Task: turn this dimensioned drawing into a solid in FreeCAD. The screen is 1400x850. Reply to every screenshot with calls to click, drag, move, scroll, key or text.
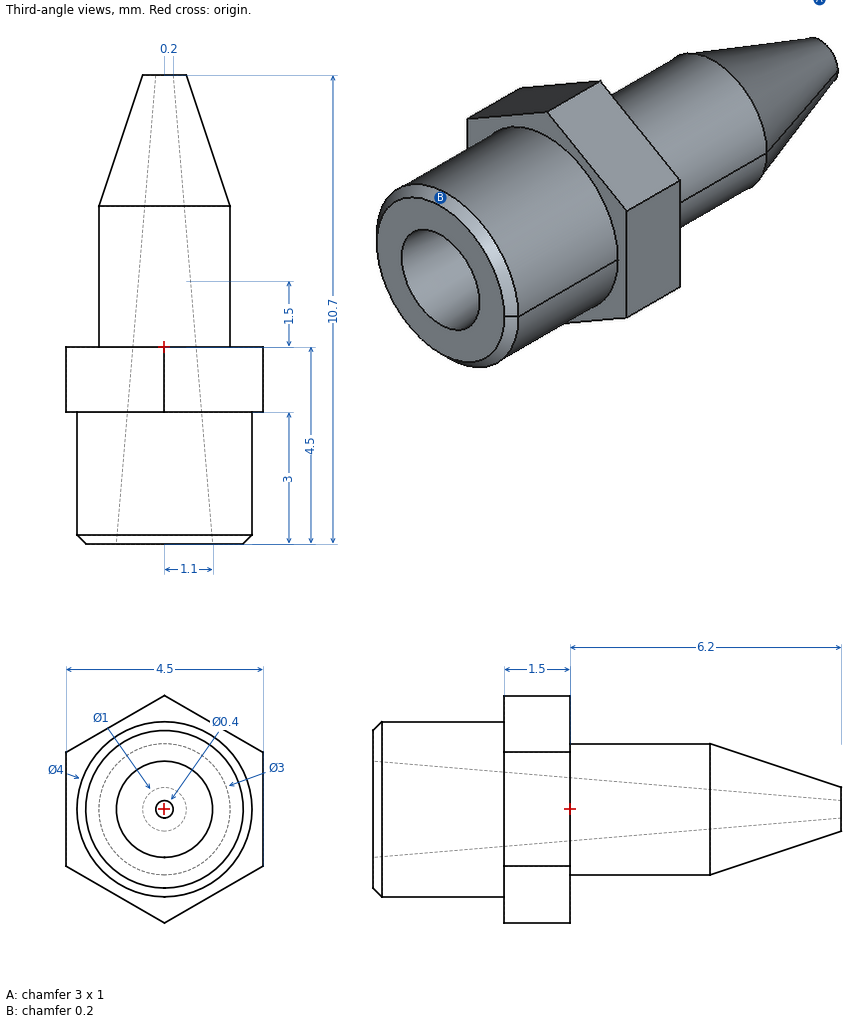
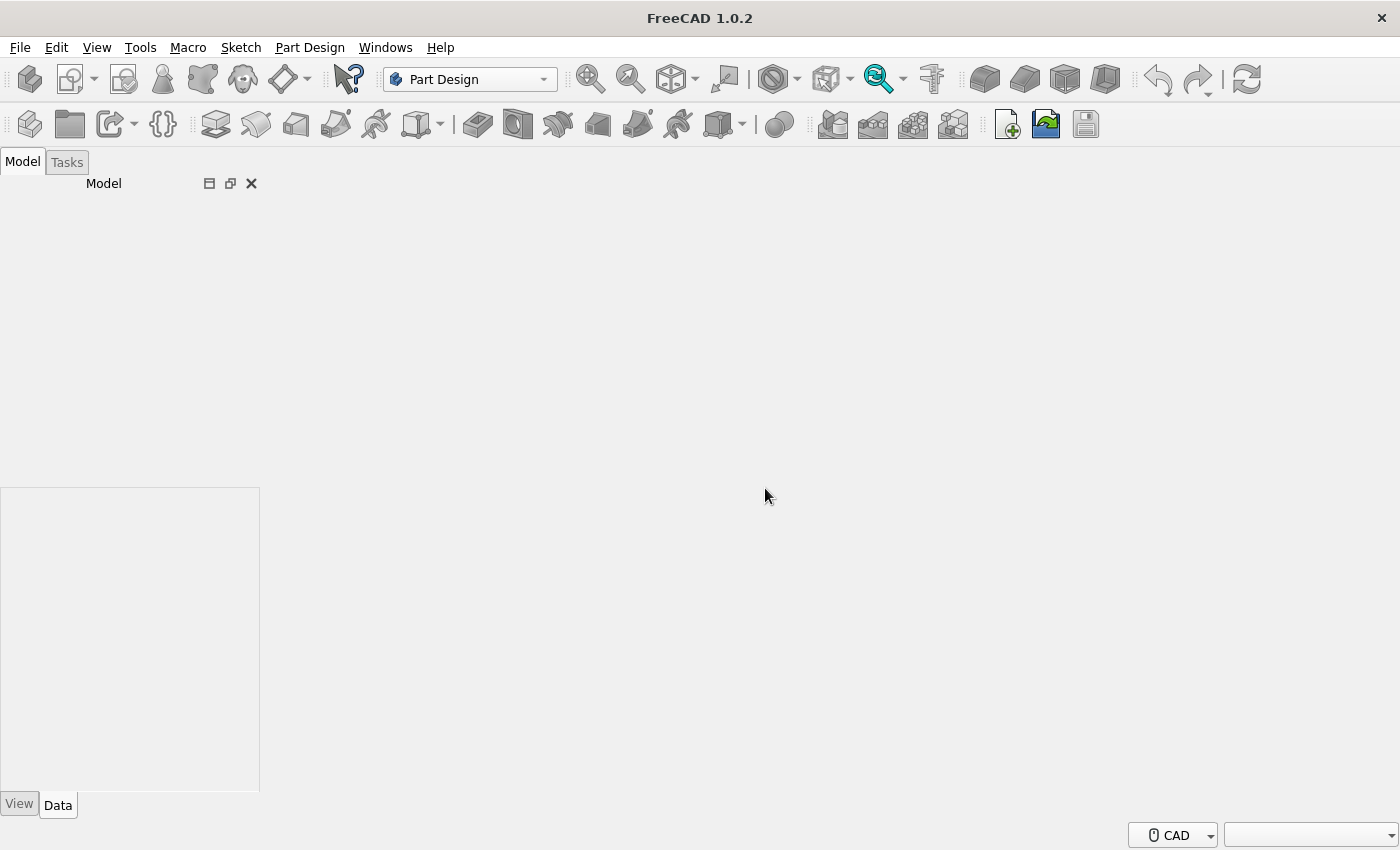
key(ctrl+n)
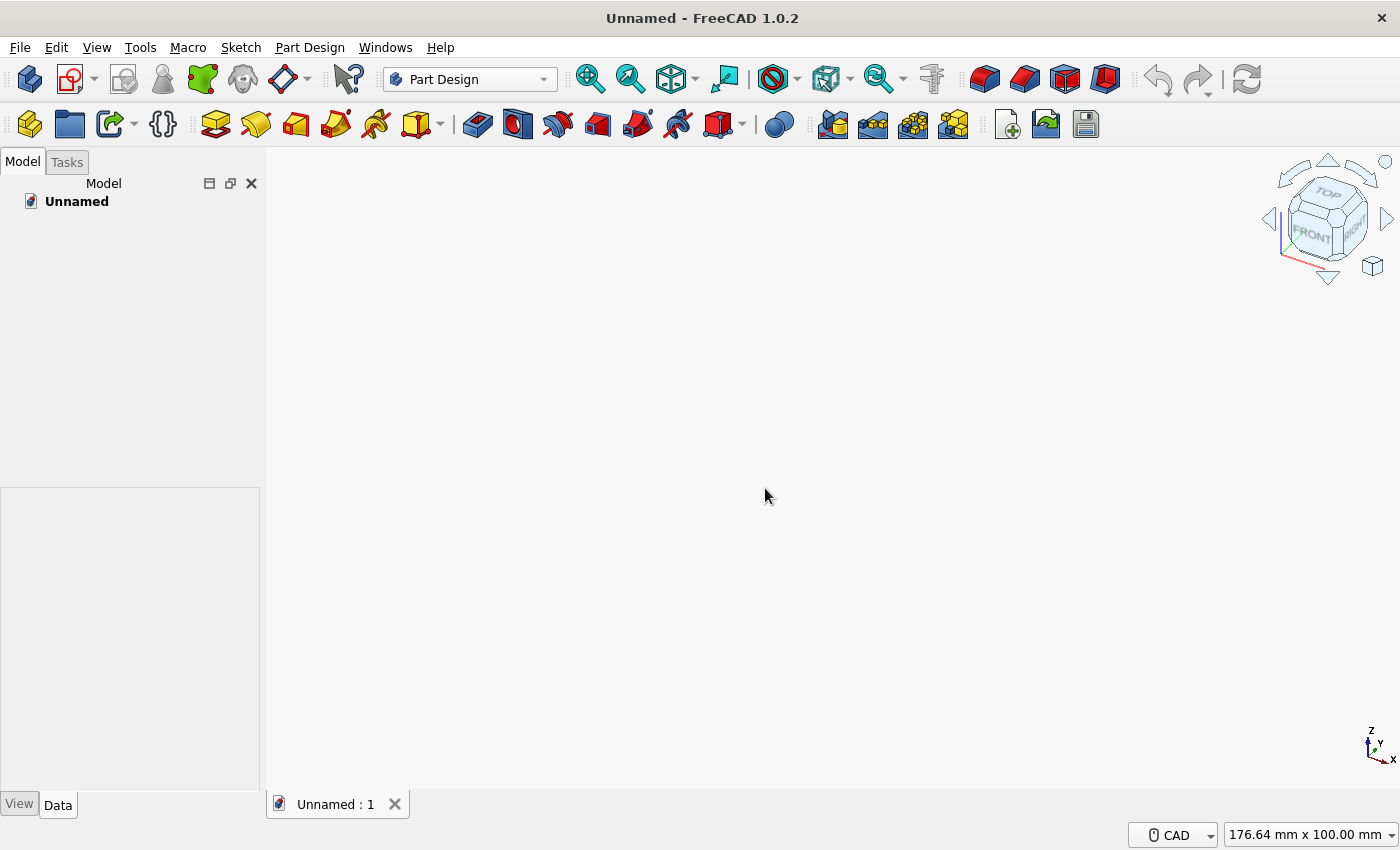
click(70, 80)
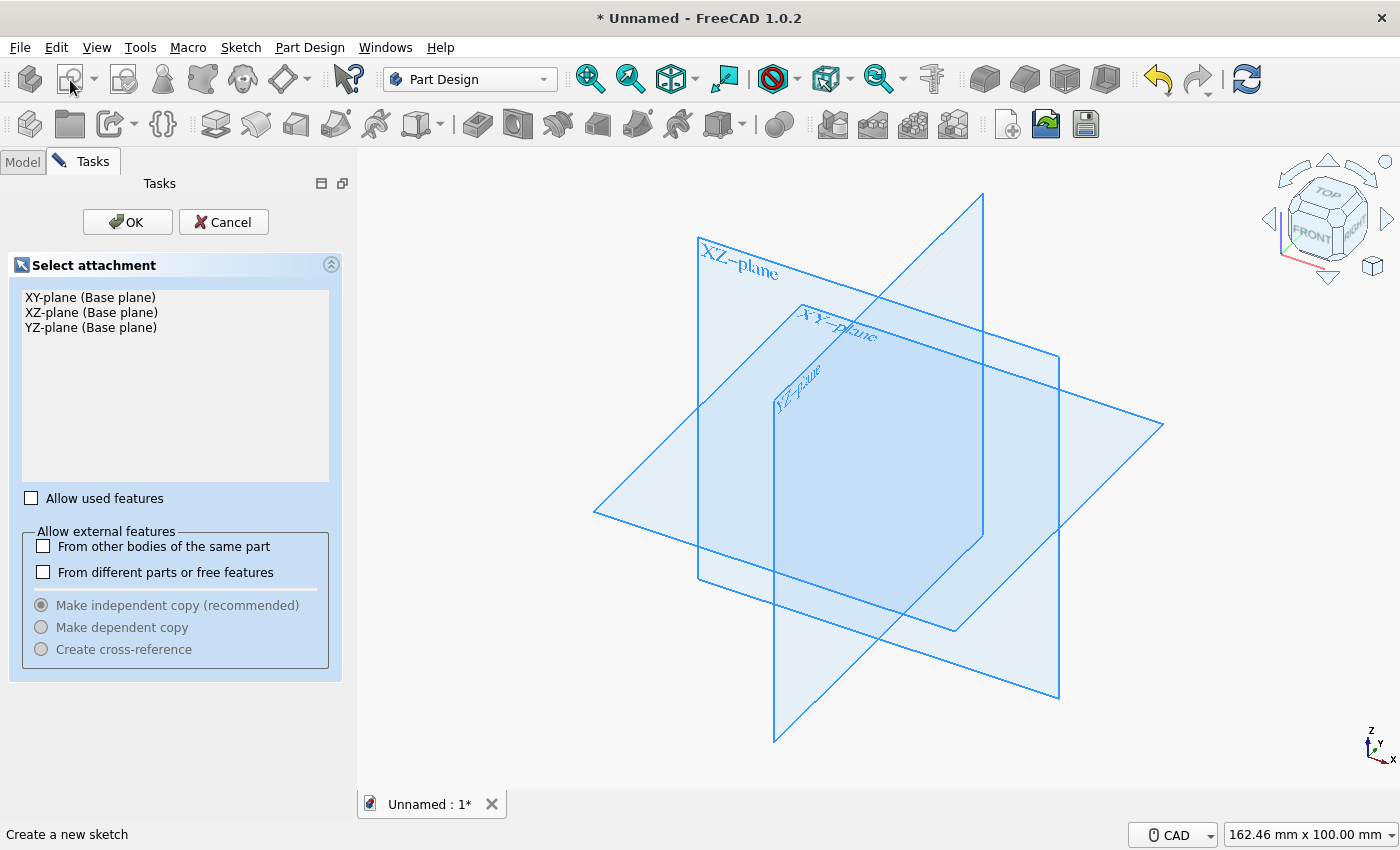
click(82, 312)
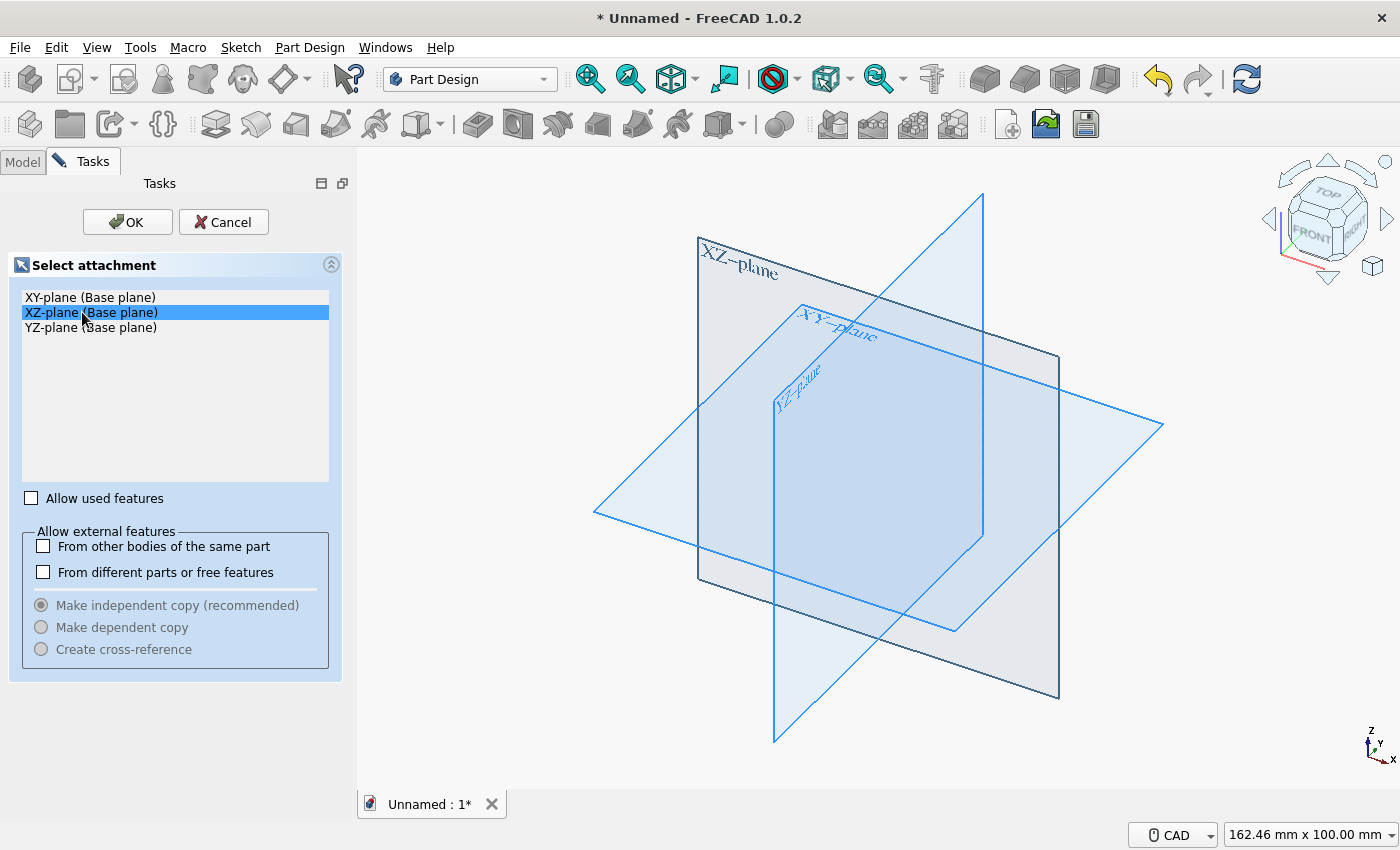
click(128, 222)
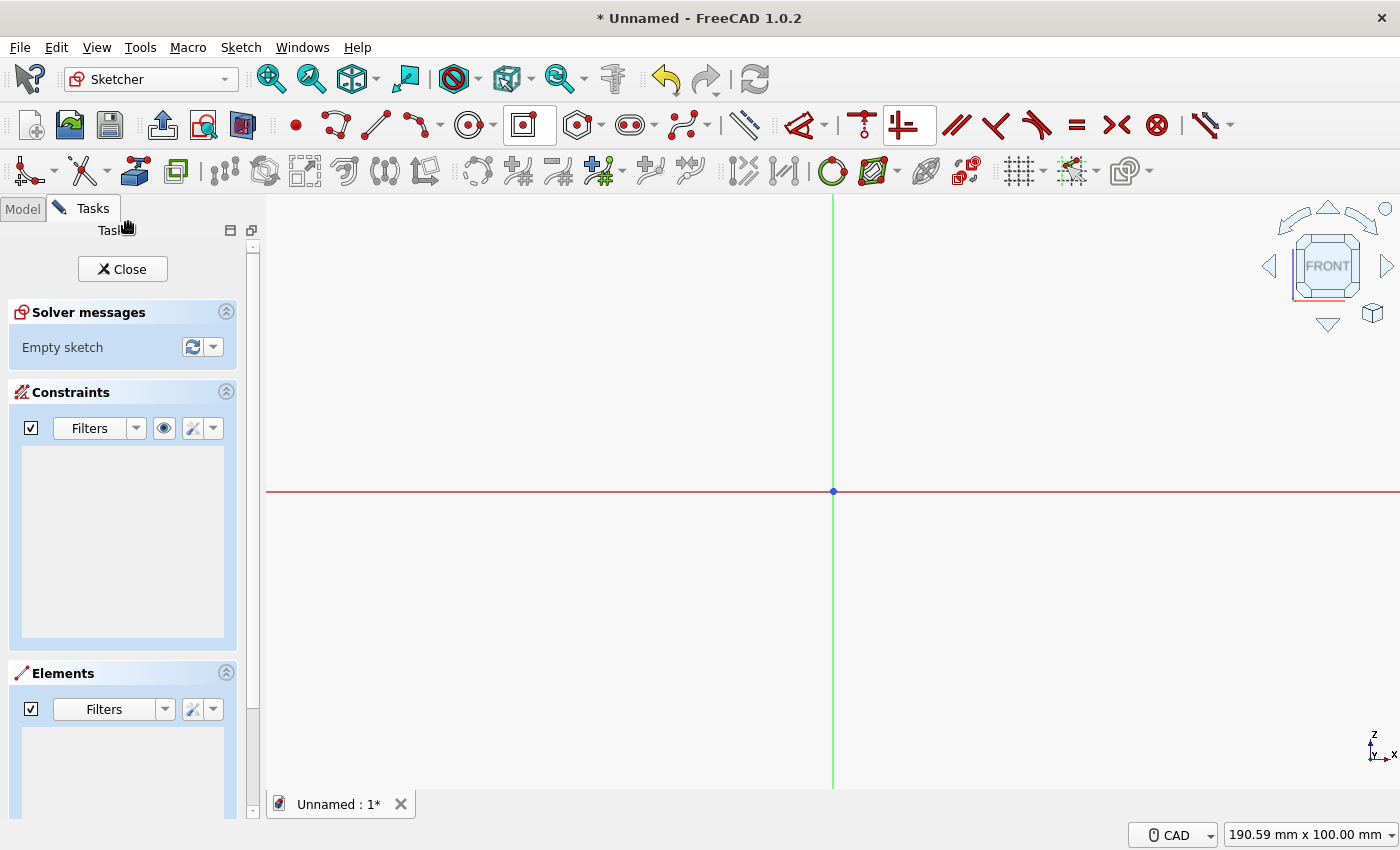
scroll(837, 492, up, 15)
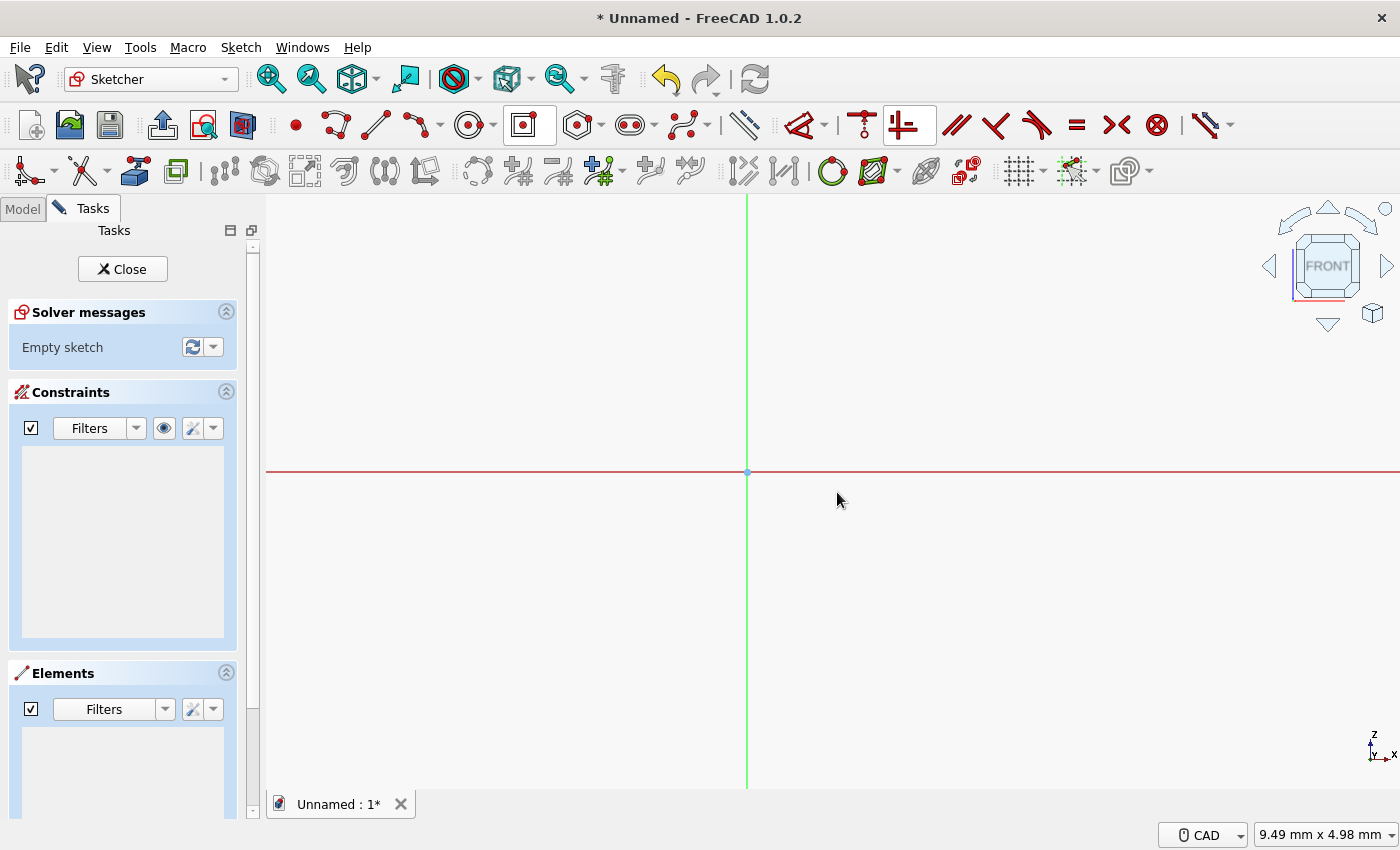
click(470, 126)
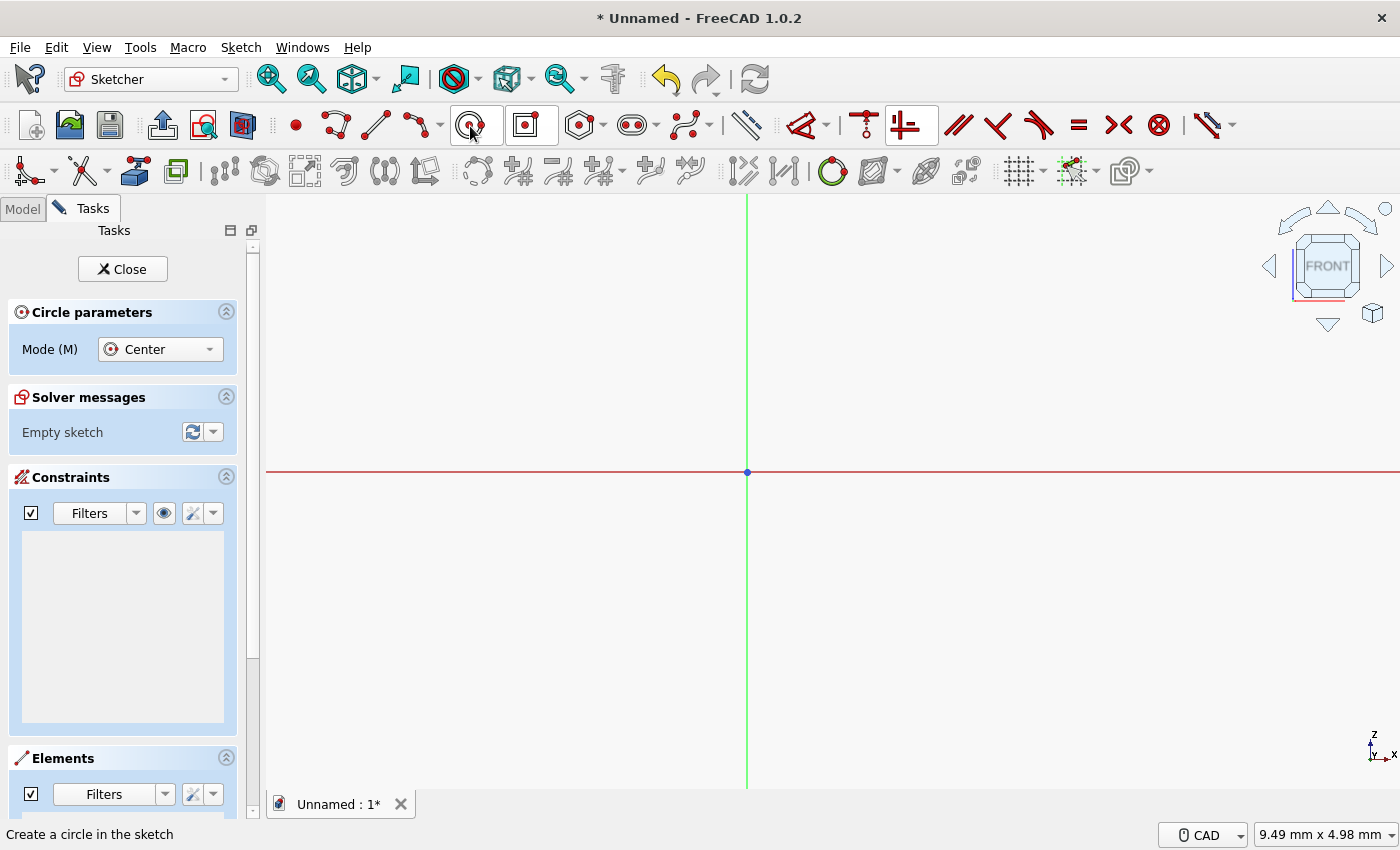
click(747, 472)
click(874, 346)
key(Escape)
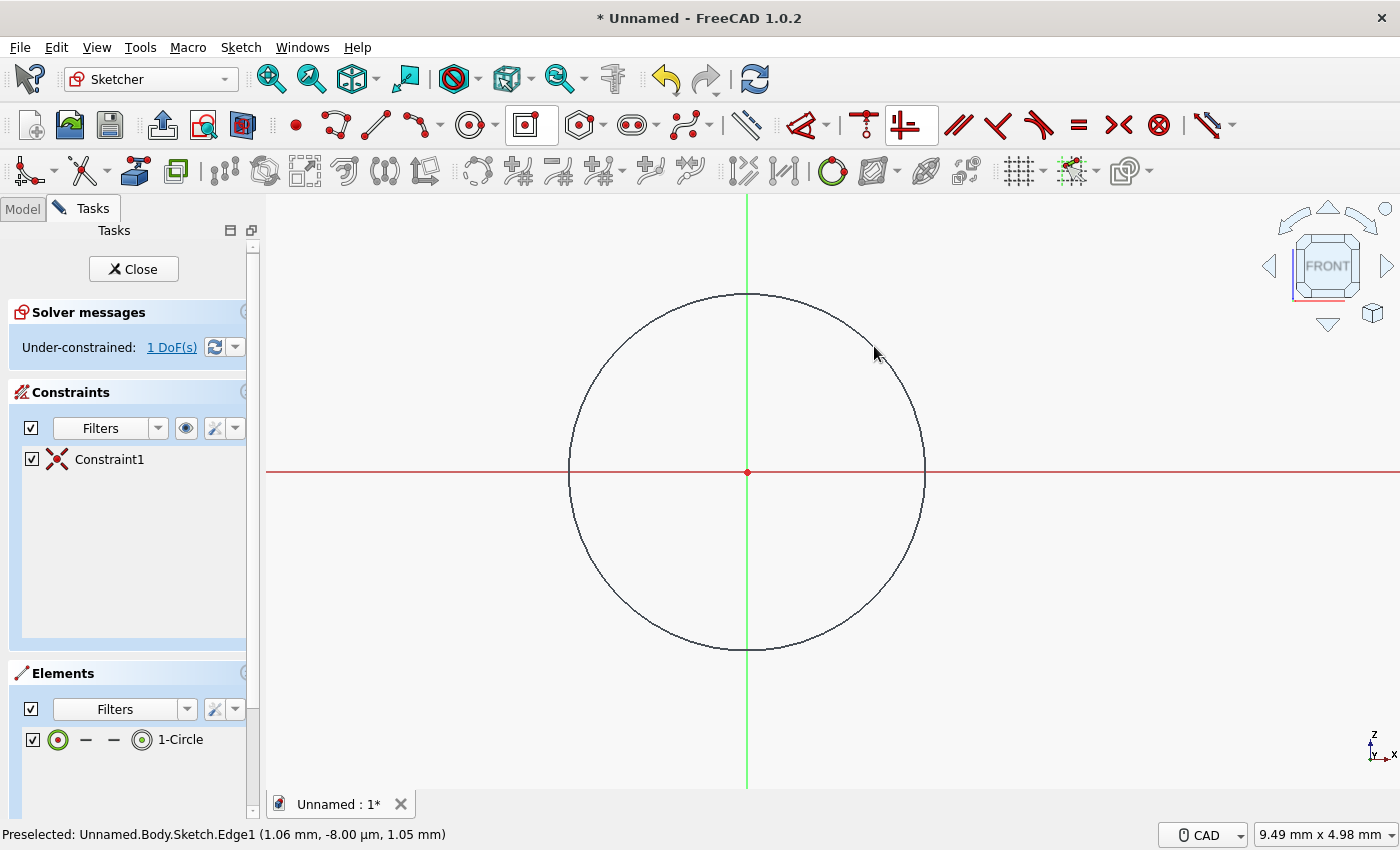
click(873, 346)